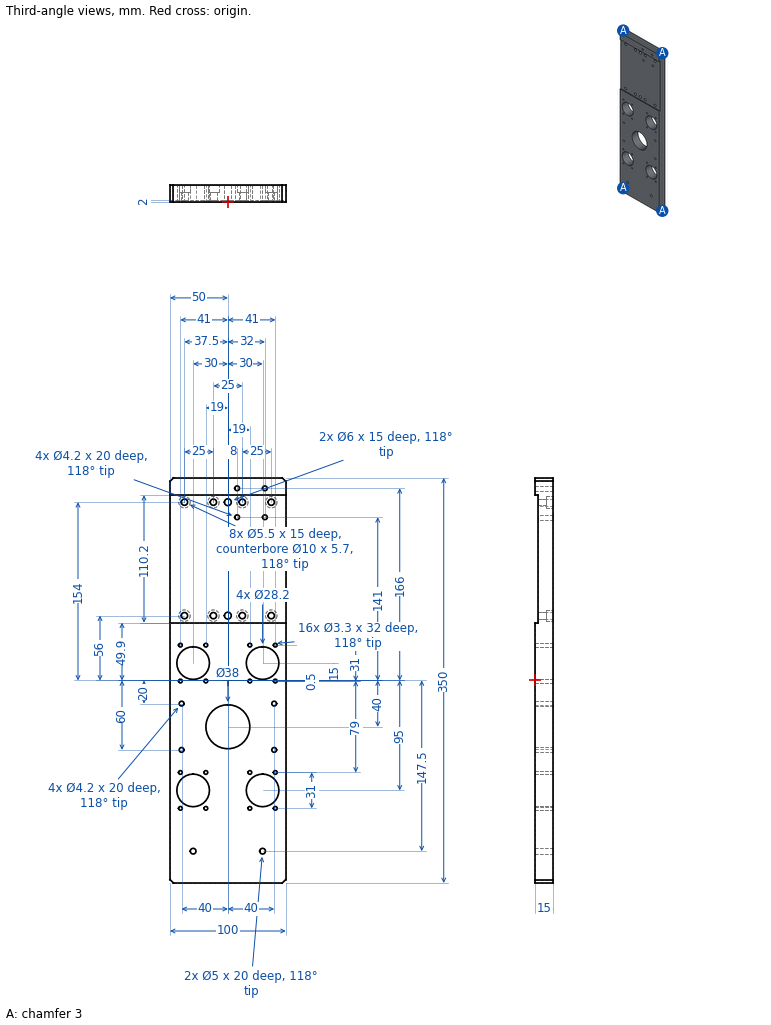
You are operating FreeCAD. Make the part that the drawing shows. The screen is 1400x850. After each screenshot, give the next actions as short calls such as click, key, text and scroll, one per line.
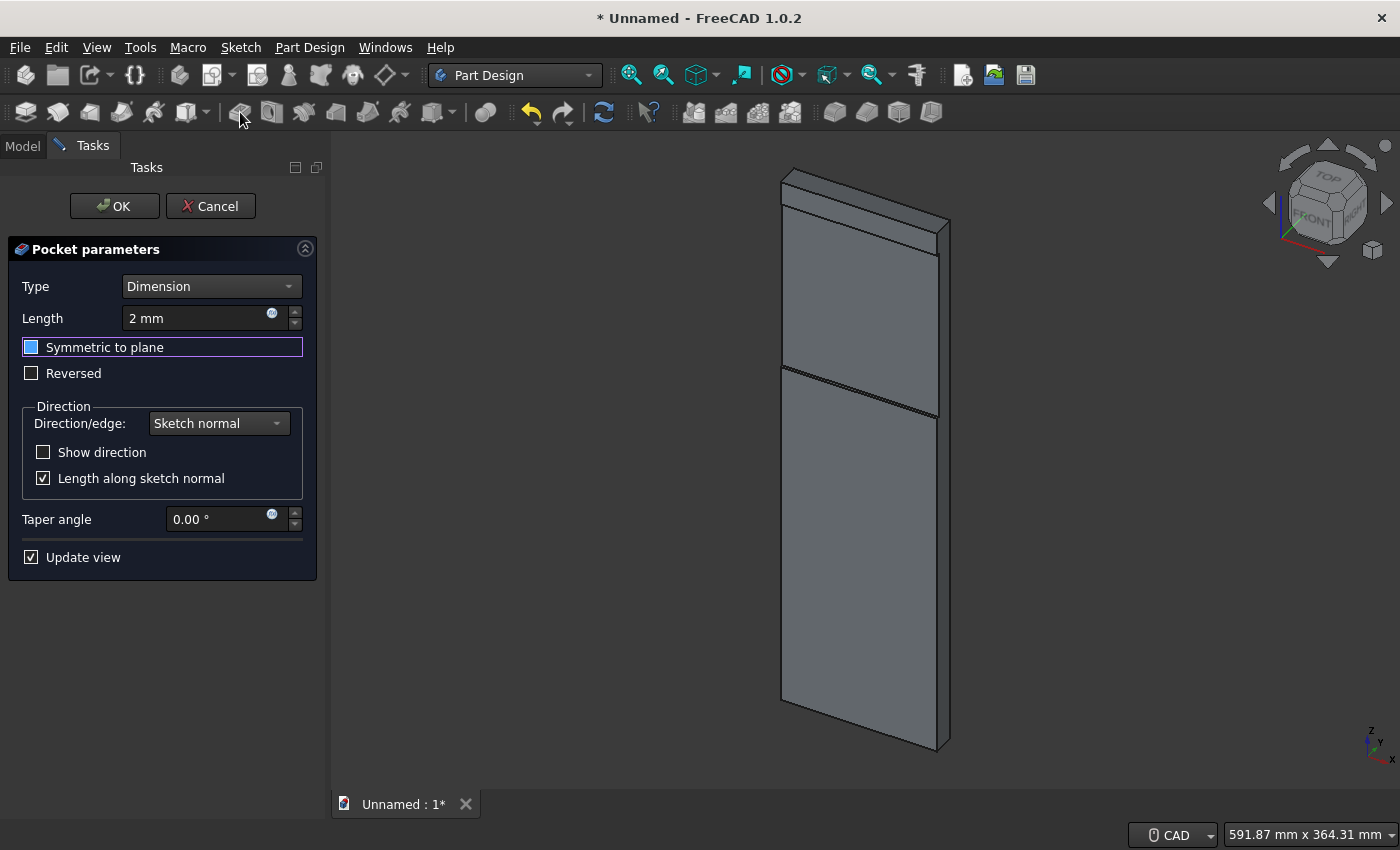
click(115, 206)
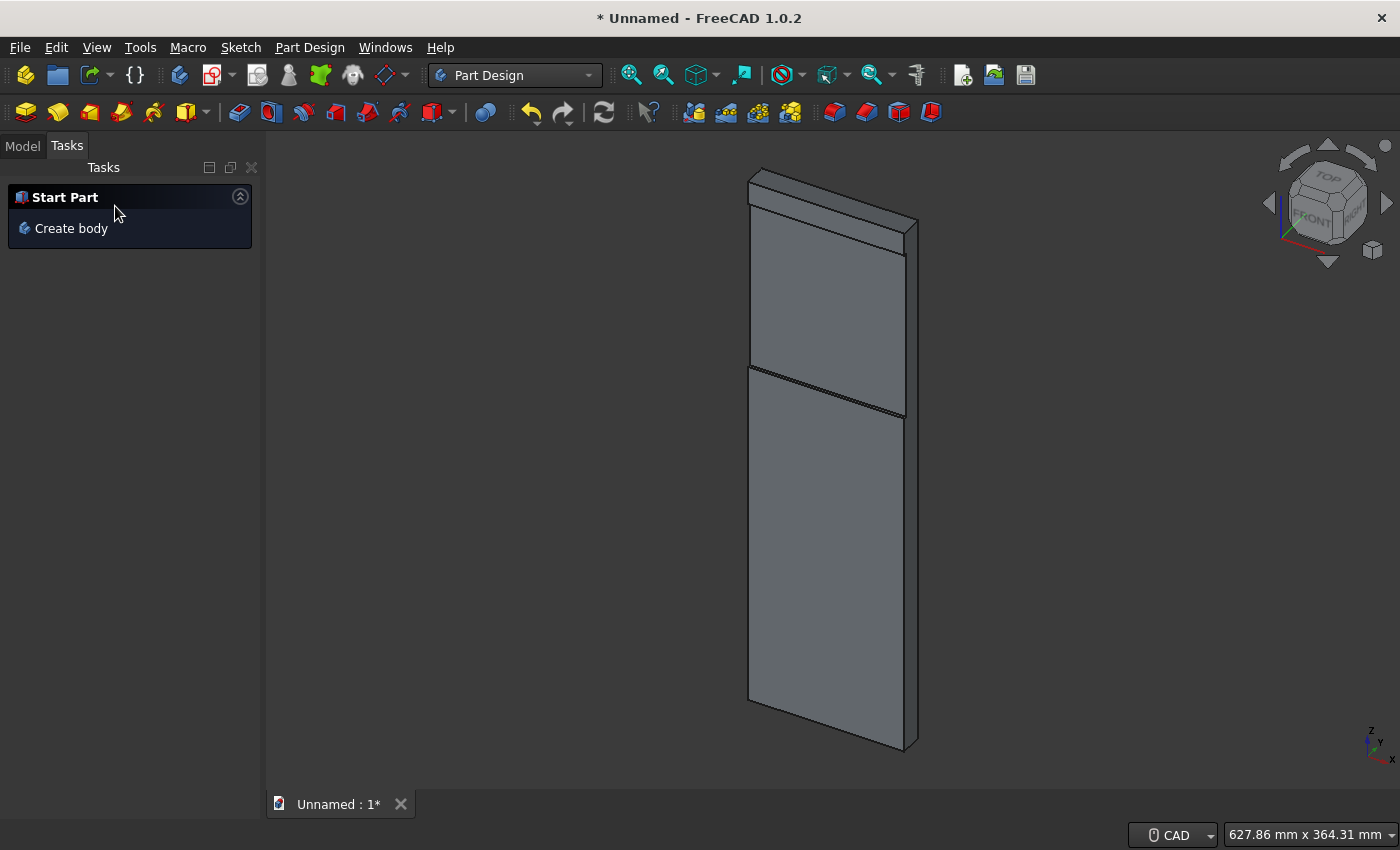
key(4)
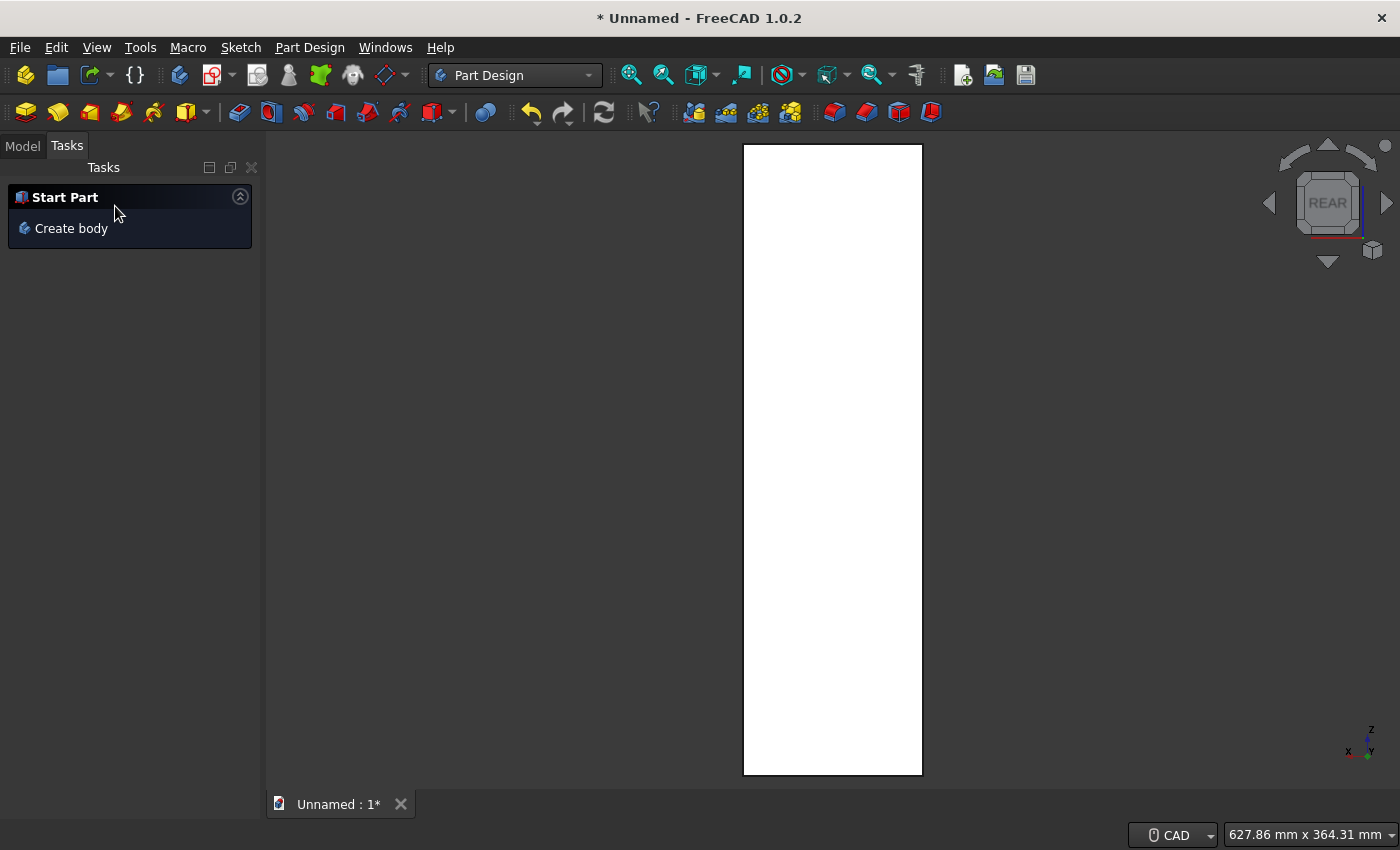
click(833, 278)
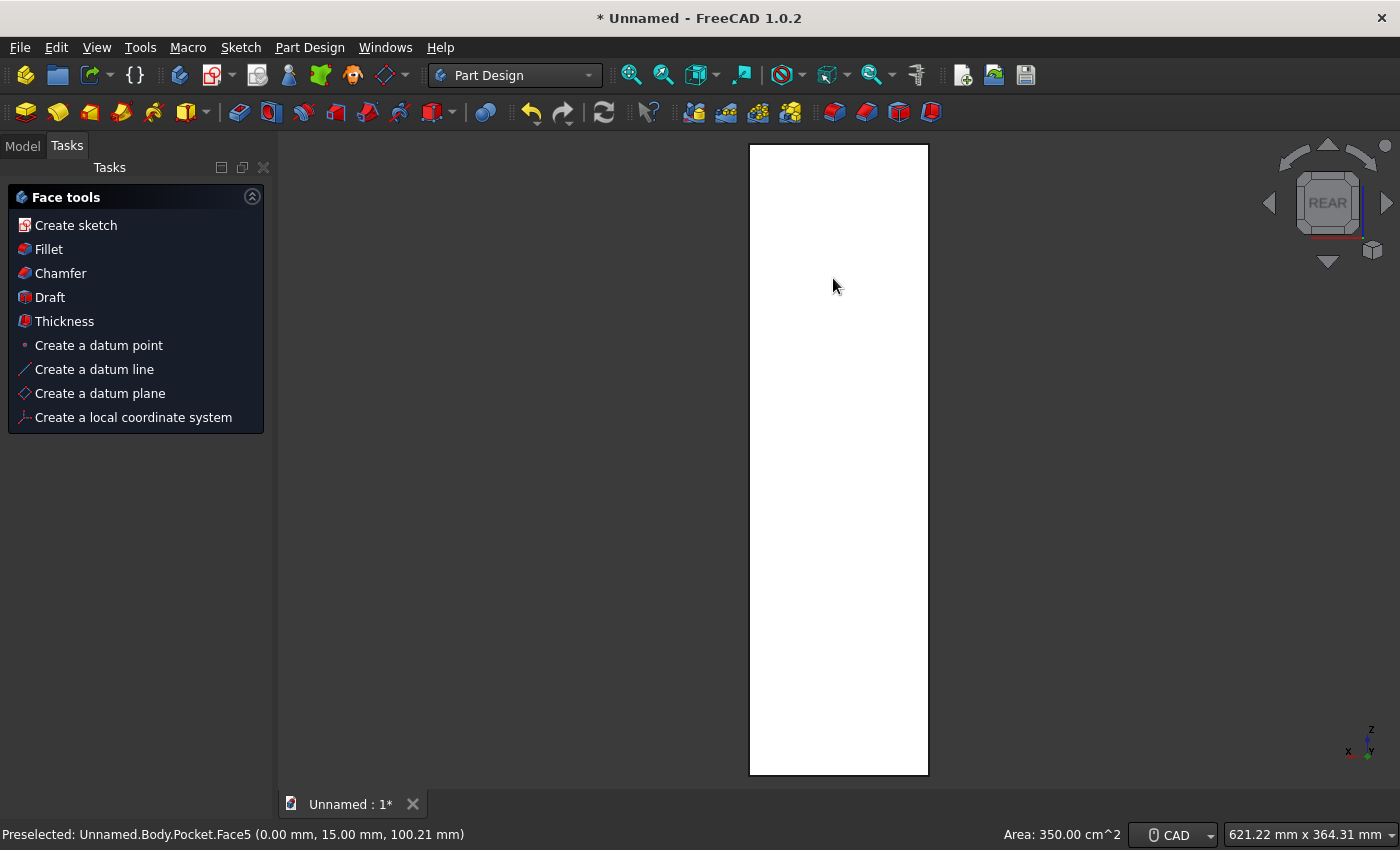
click(212, 76)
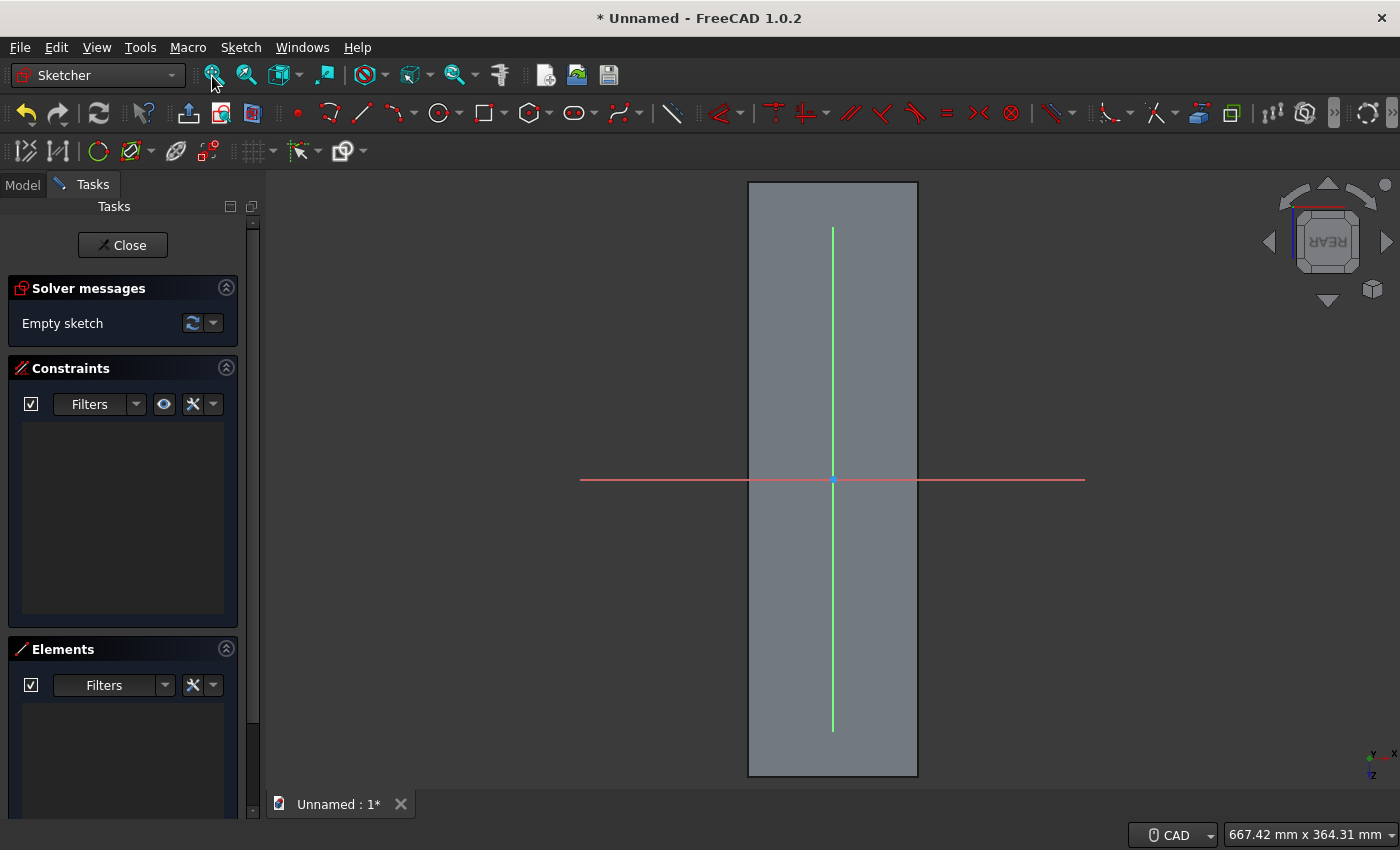
scroll(455, 198, down, 1)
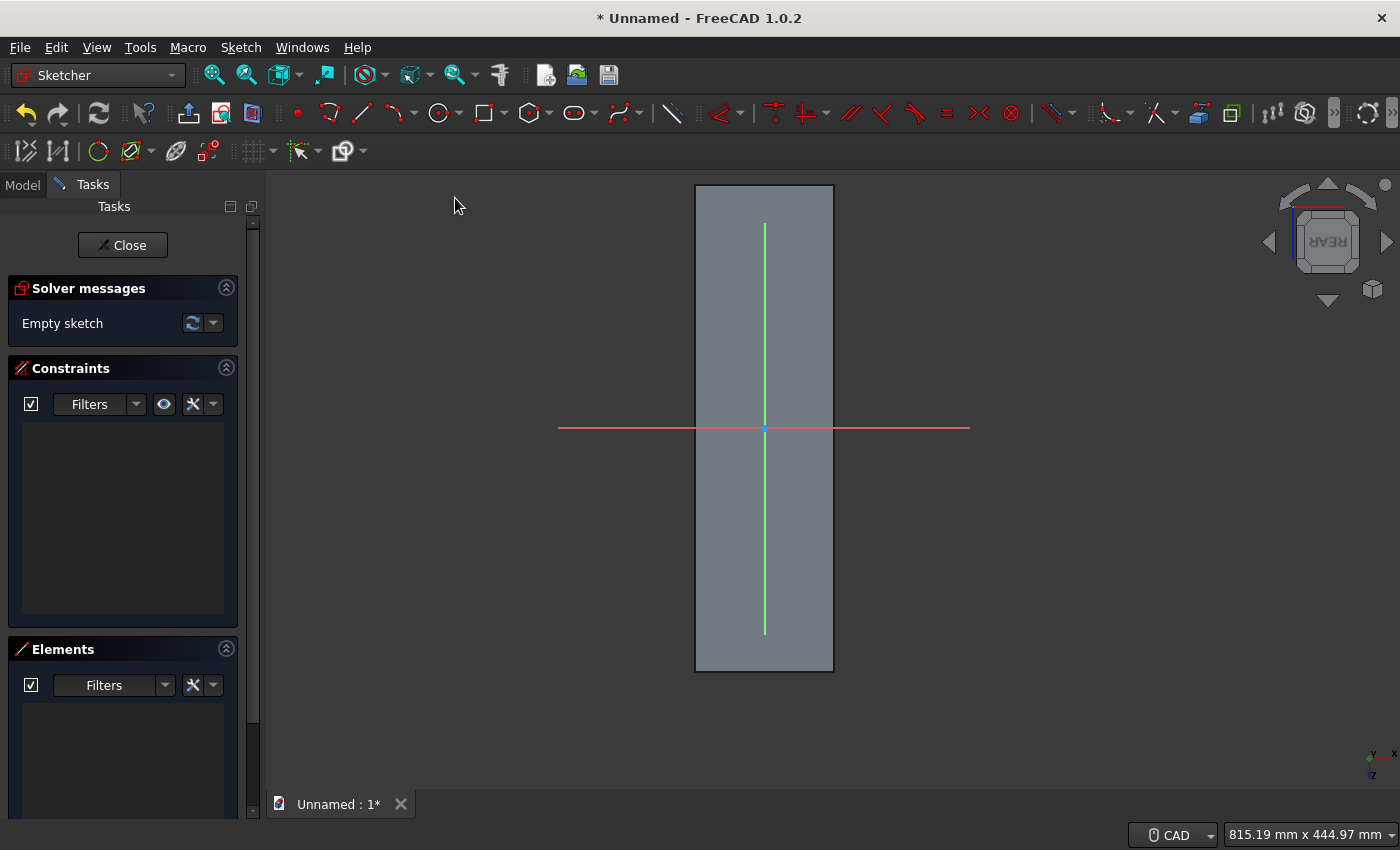
scroll(765, 608, up, 3)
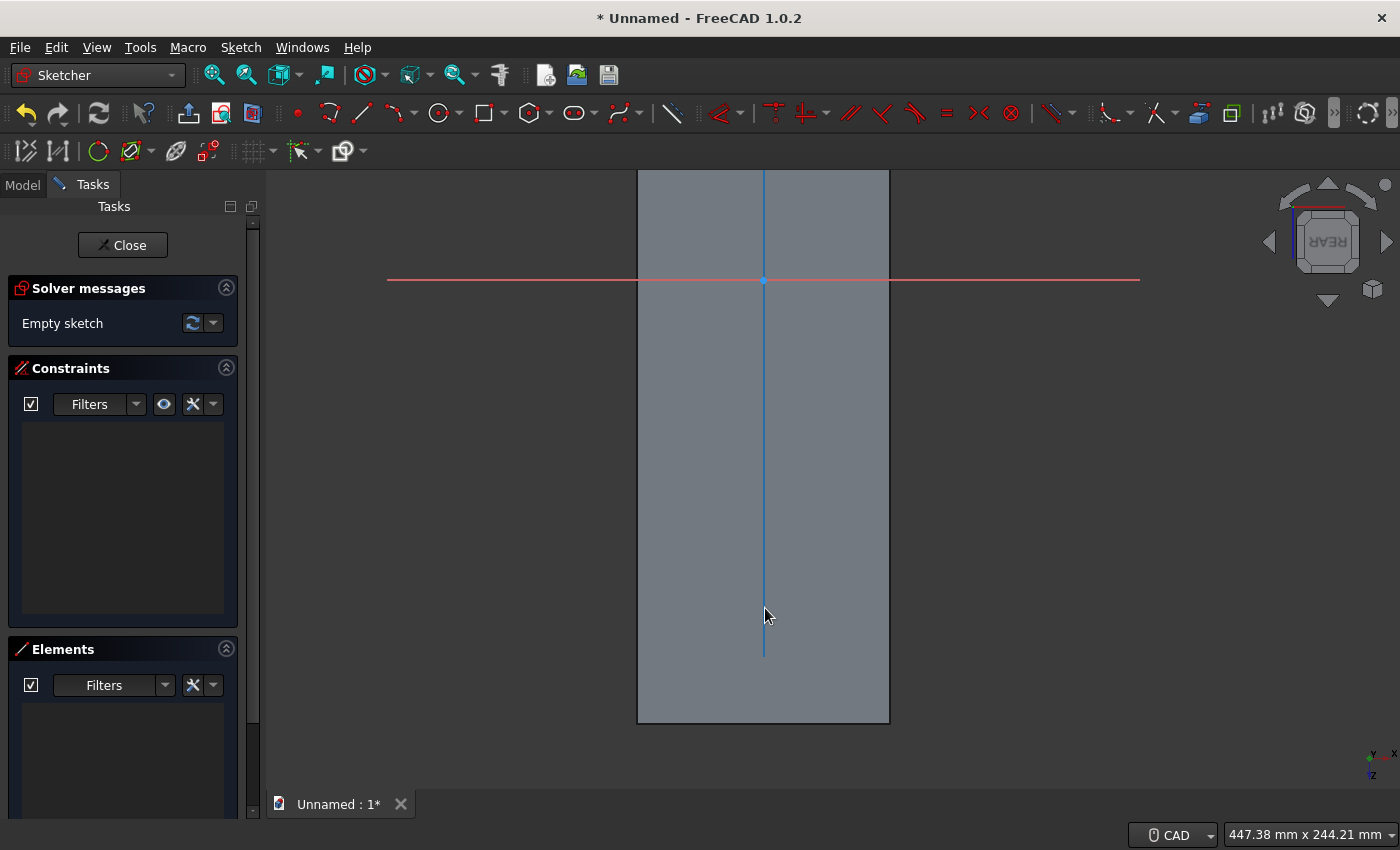
key(g)
key(c)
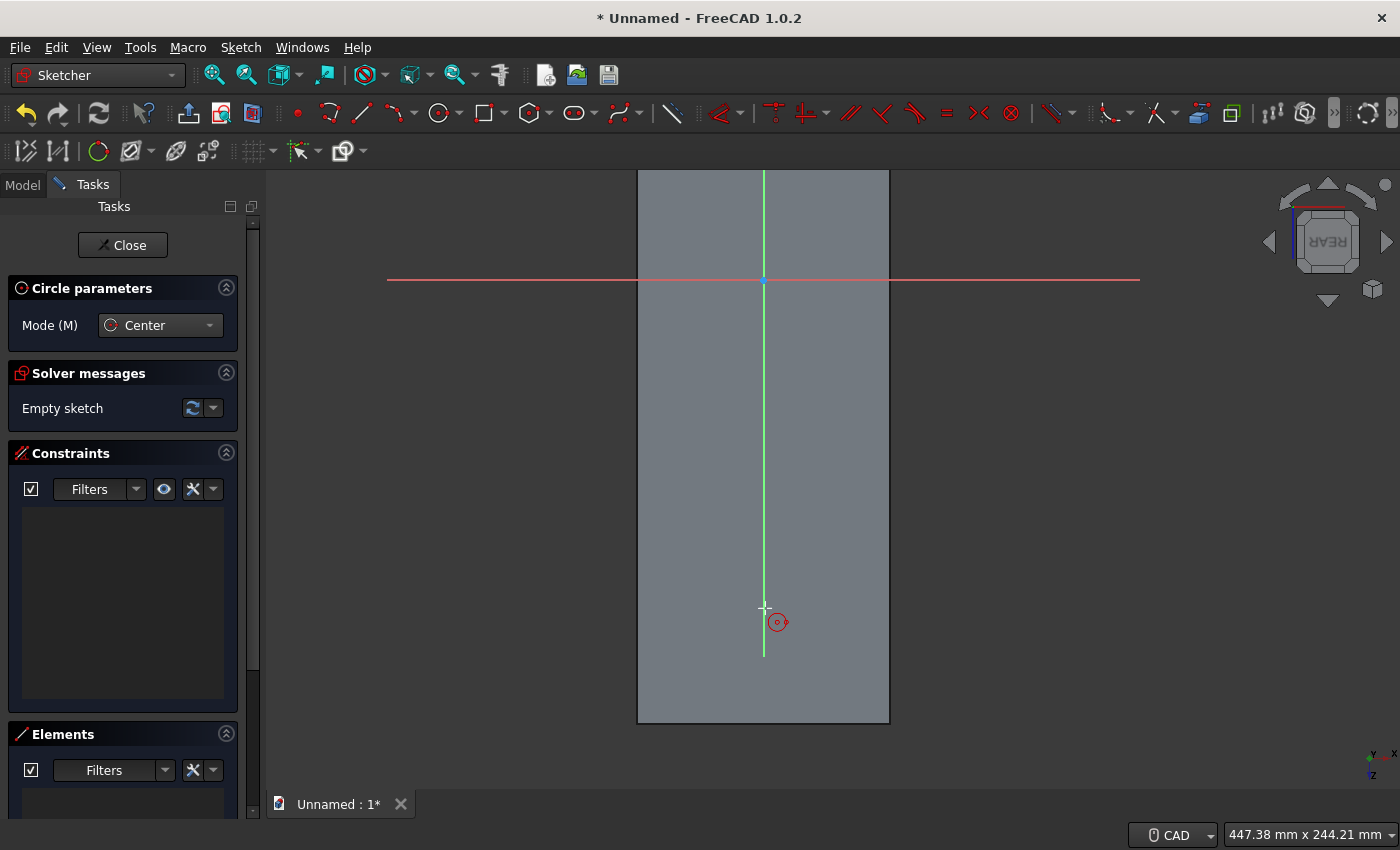
scroll(669, 671, up, 6)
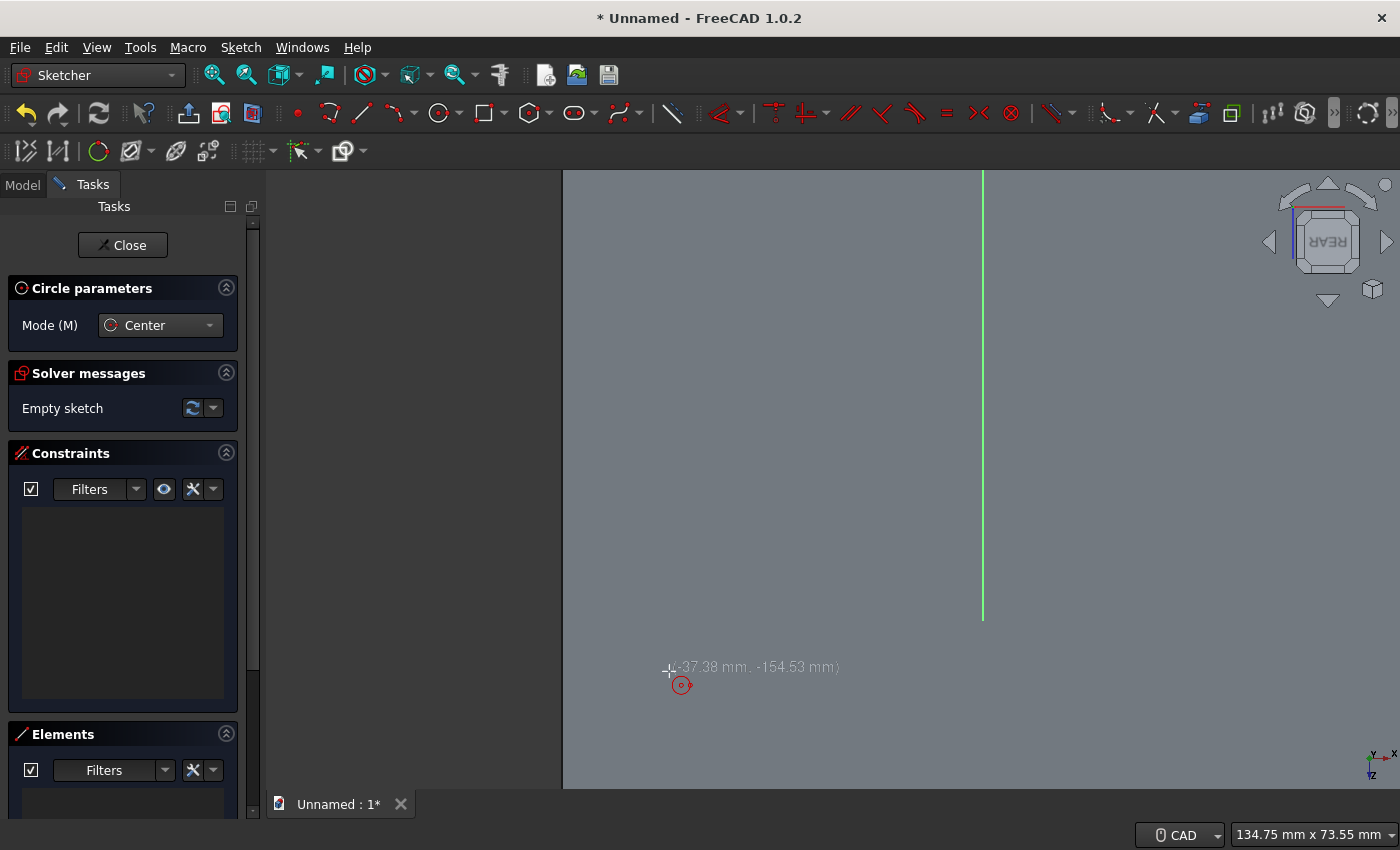
click(667, 668)
click(684, 652)